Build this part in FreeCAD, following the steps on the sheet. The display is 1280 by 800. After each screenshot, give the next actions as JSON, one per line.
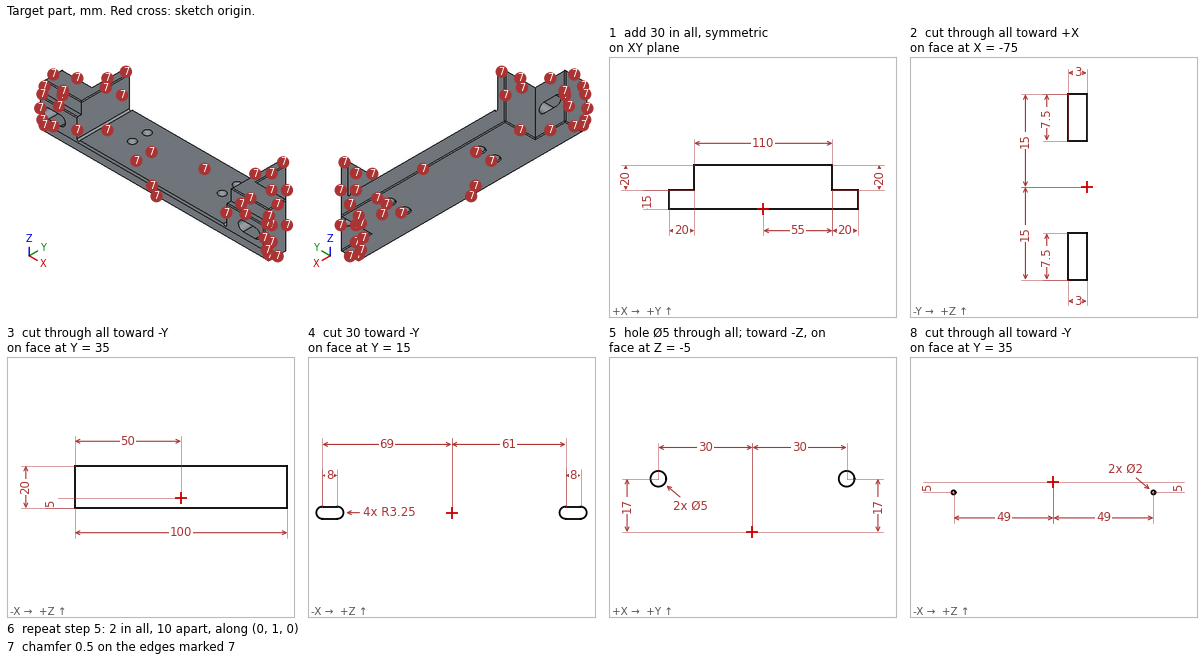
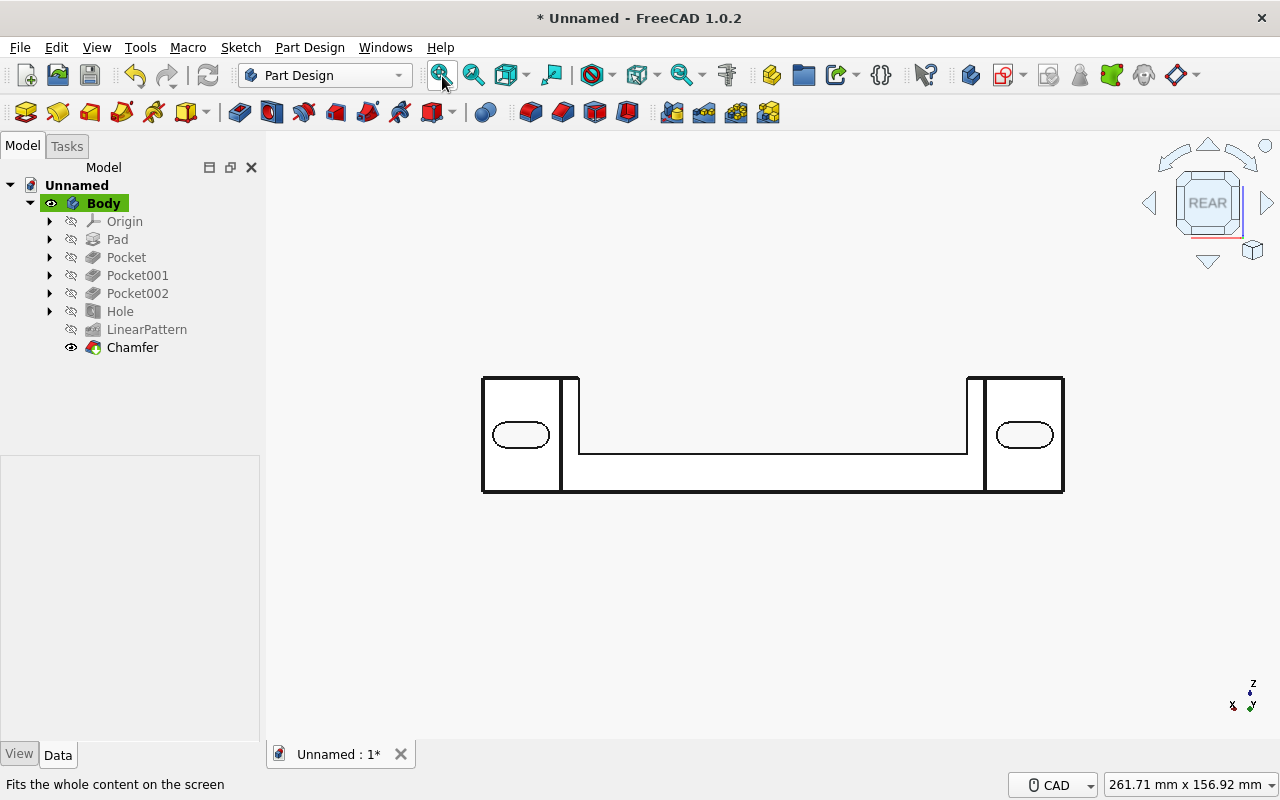
{"action": "left_click", "coordinate": [592, 466]}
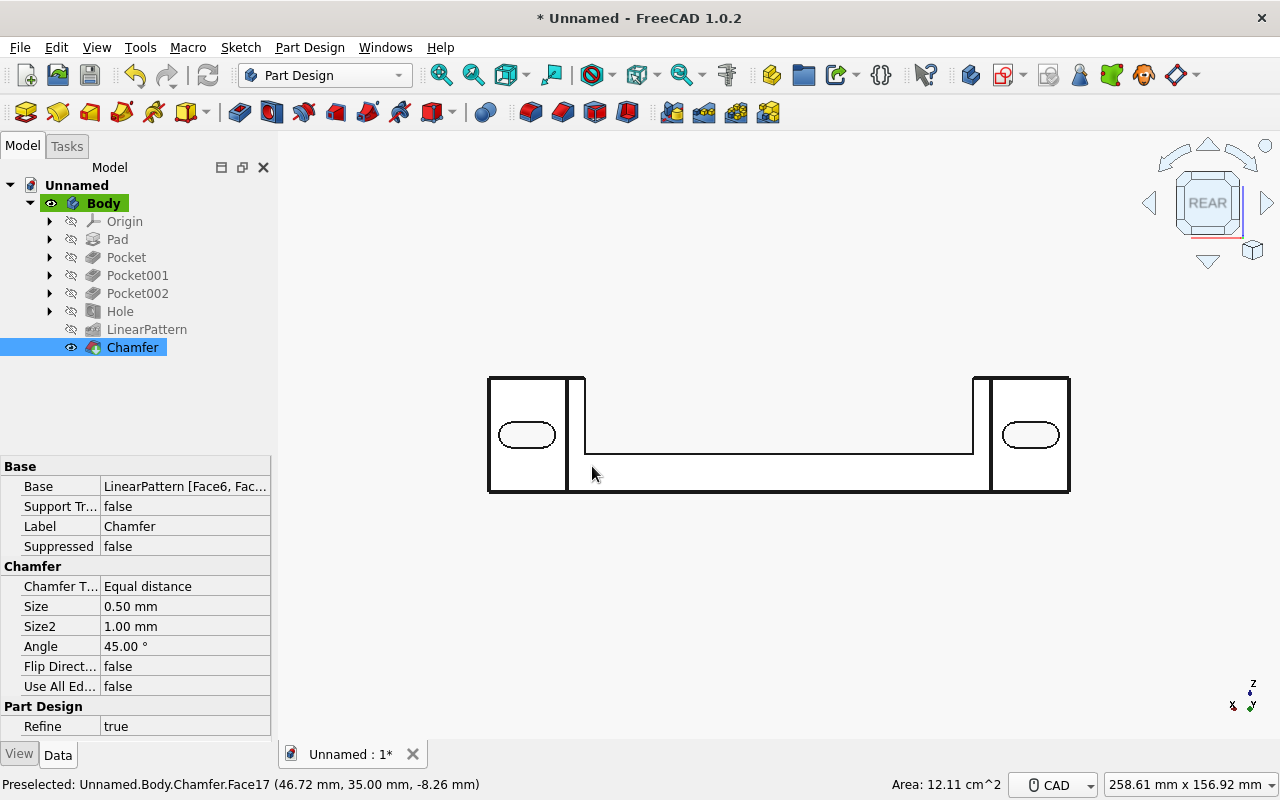
{"action": "left_click", "coordinate": [1004, 76]}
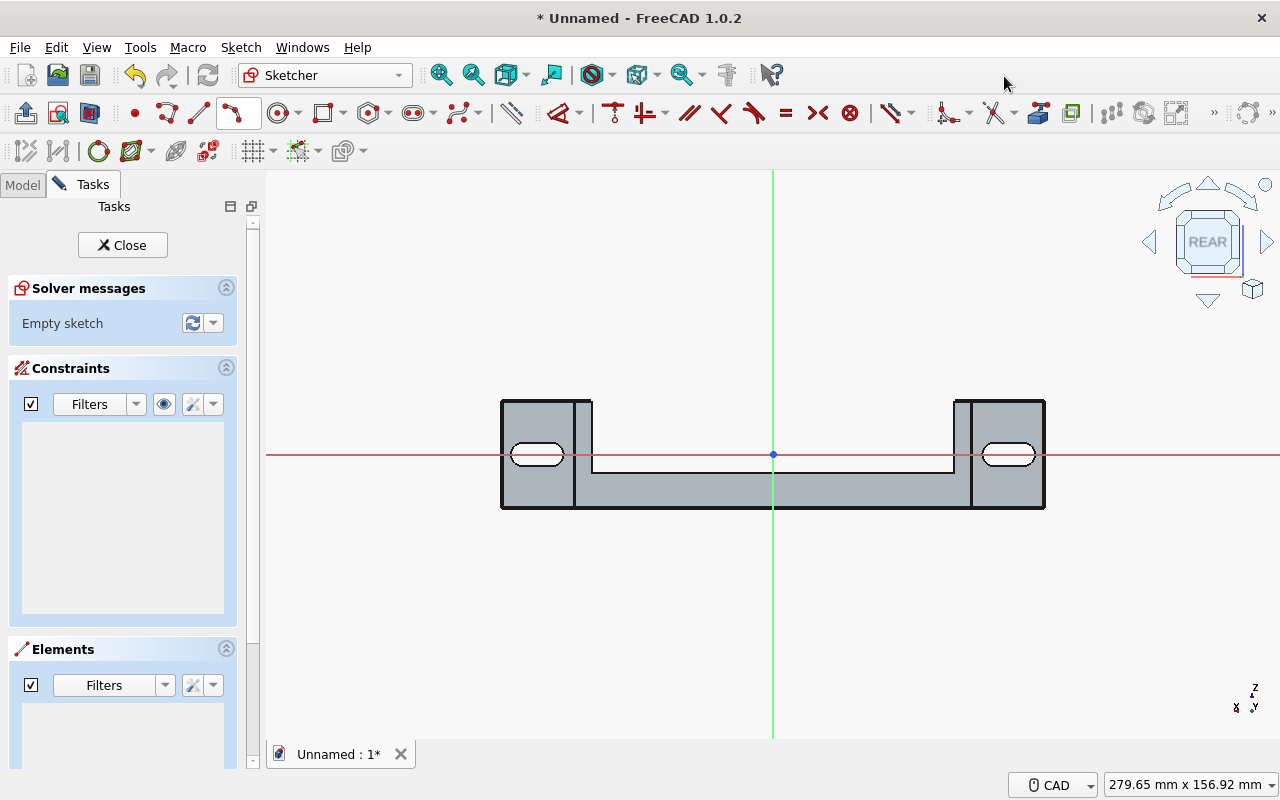
{"action": "scroll", "coordinate": [912, 487], "scroll_direction": "up", "scroll_amount": 2}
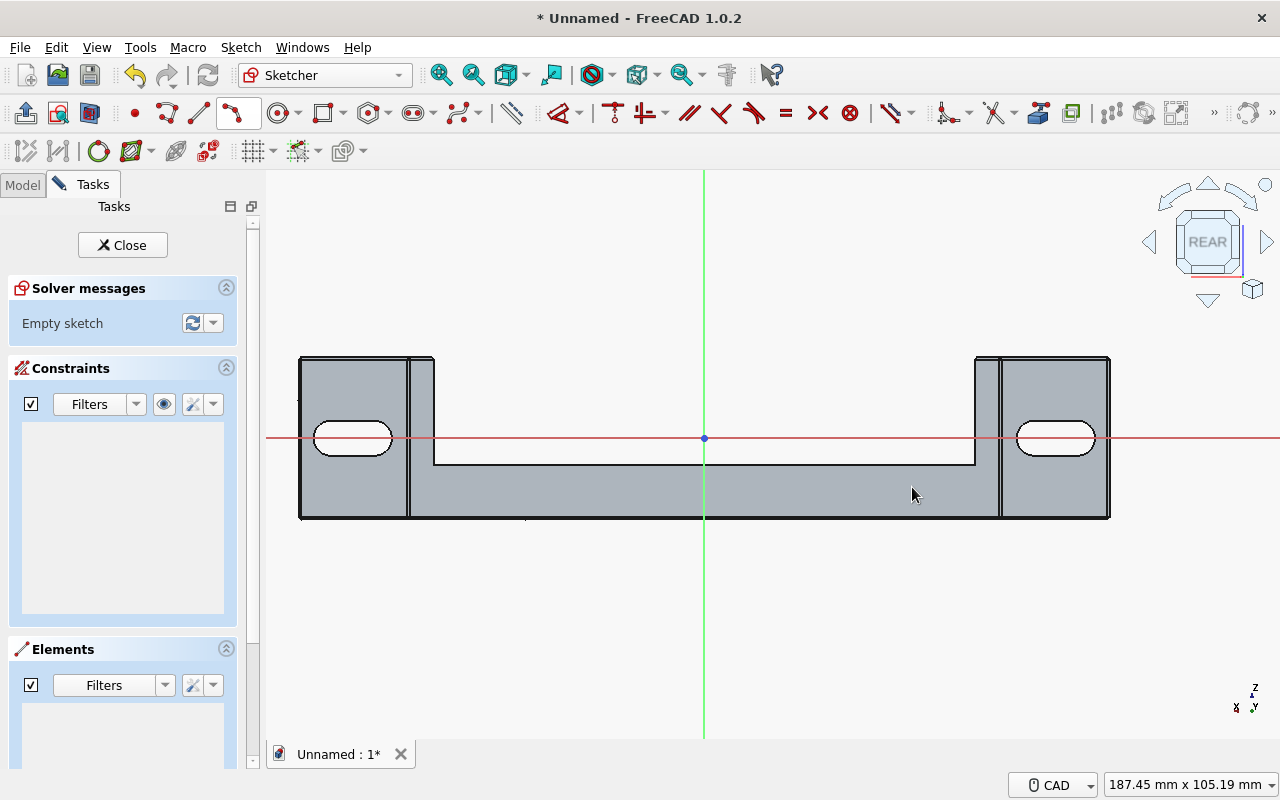
{"action": "key", "text": "g c"}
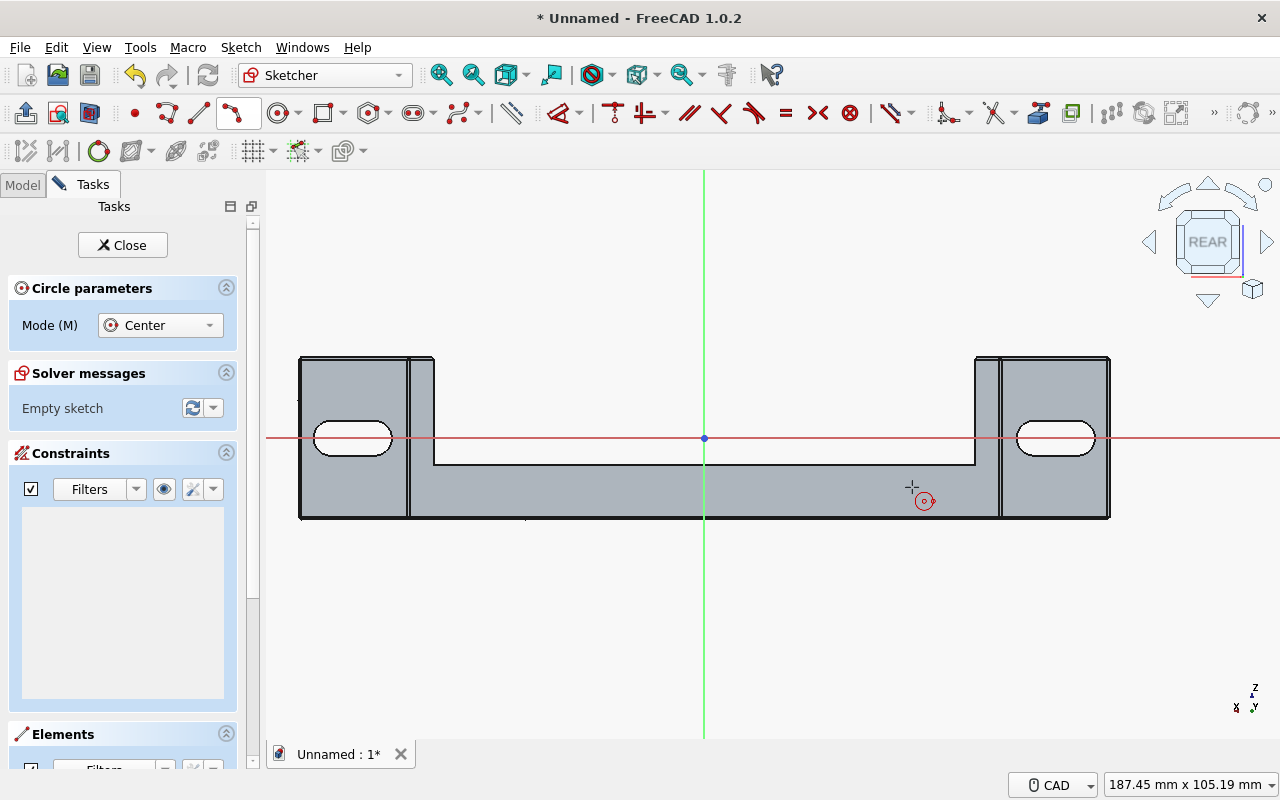
{"action": "scroll", "coordinate": [969, 465], "scroll_direction": "up", "scroll_amount": 8}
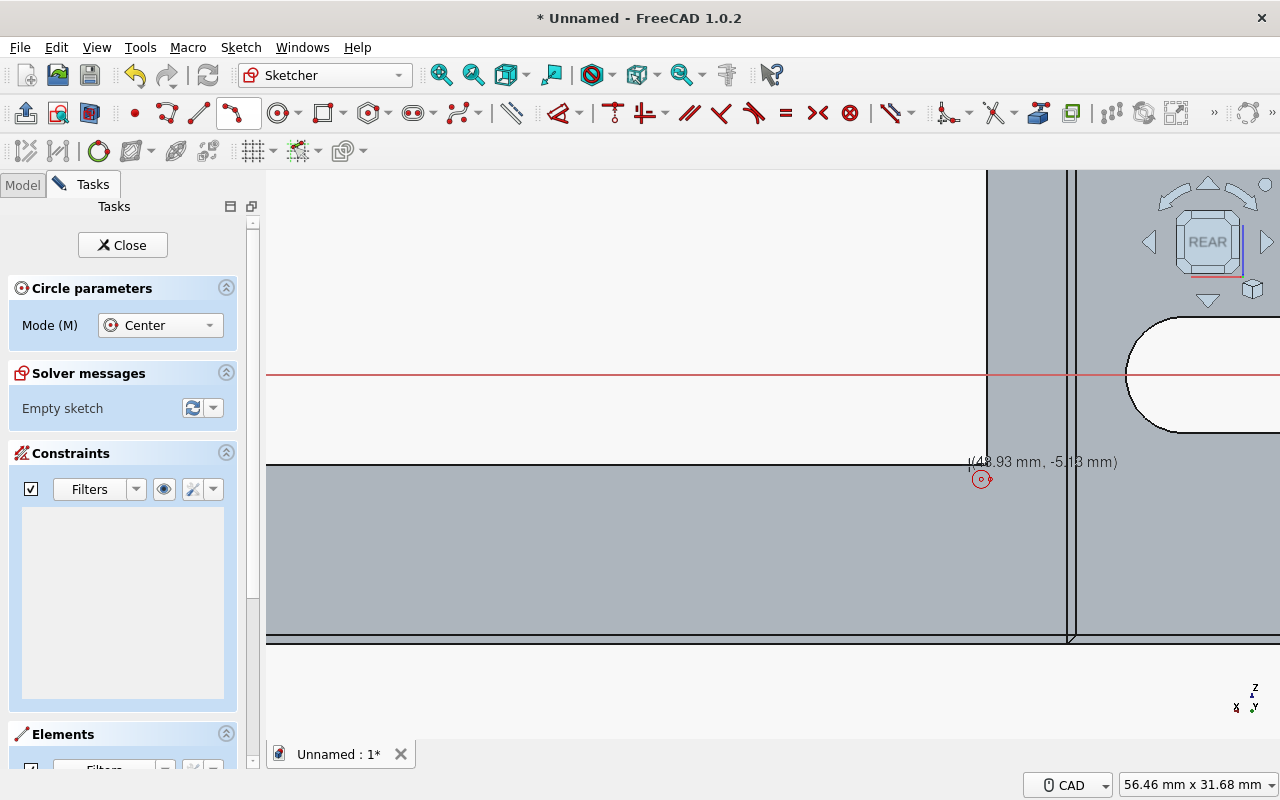
{"action": "scroll", "coordinate": [970, 466], "scroll_direction": "down", "scroll_amount": 8}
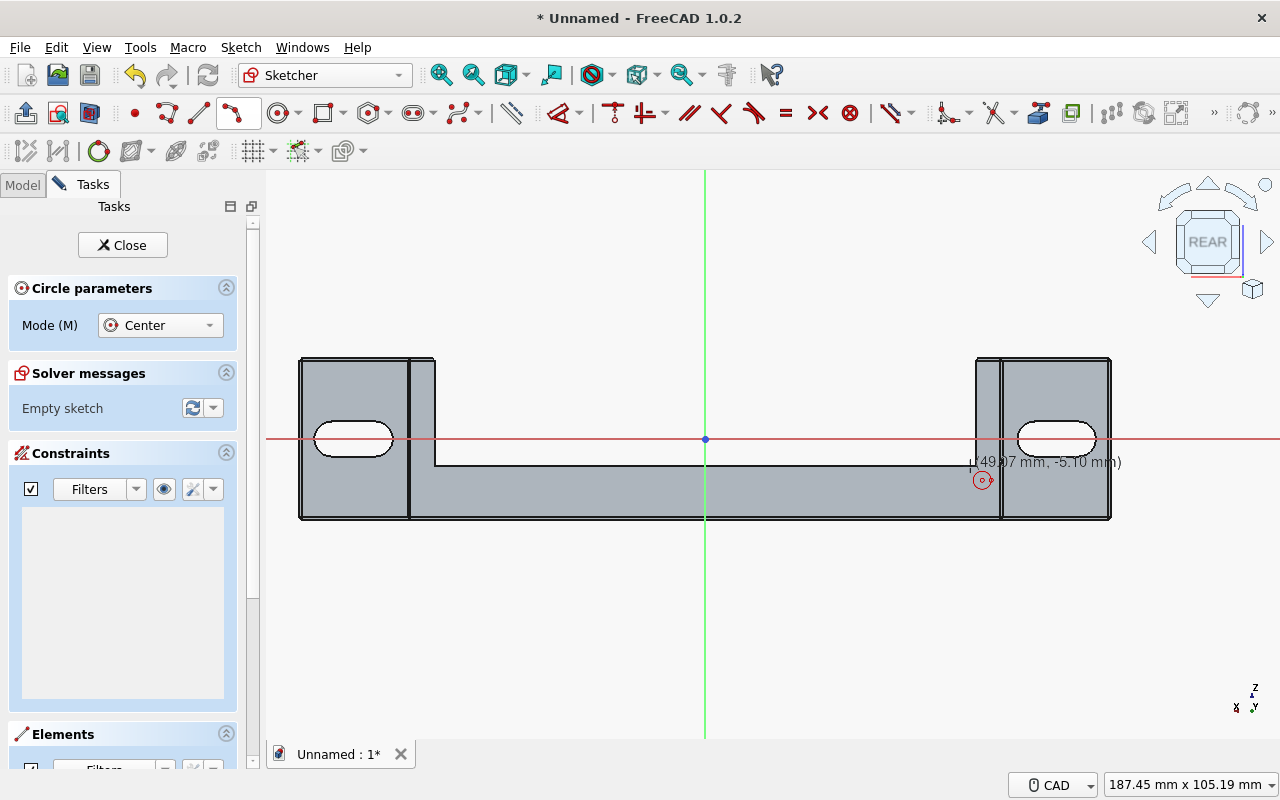
{"action": "left_click", "coordinate": [970, 466]}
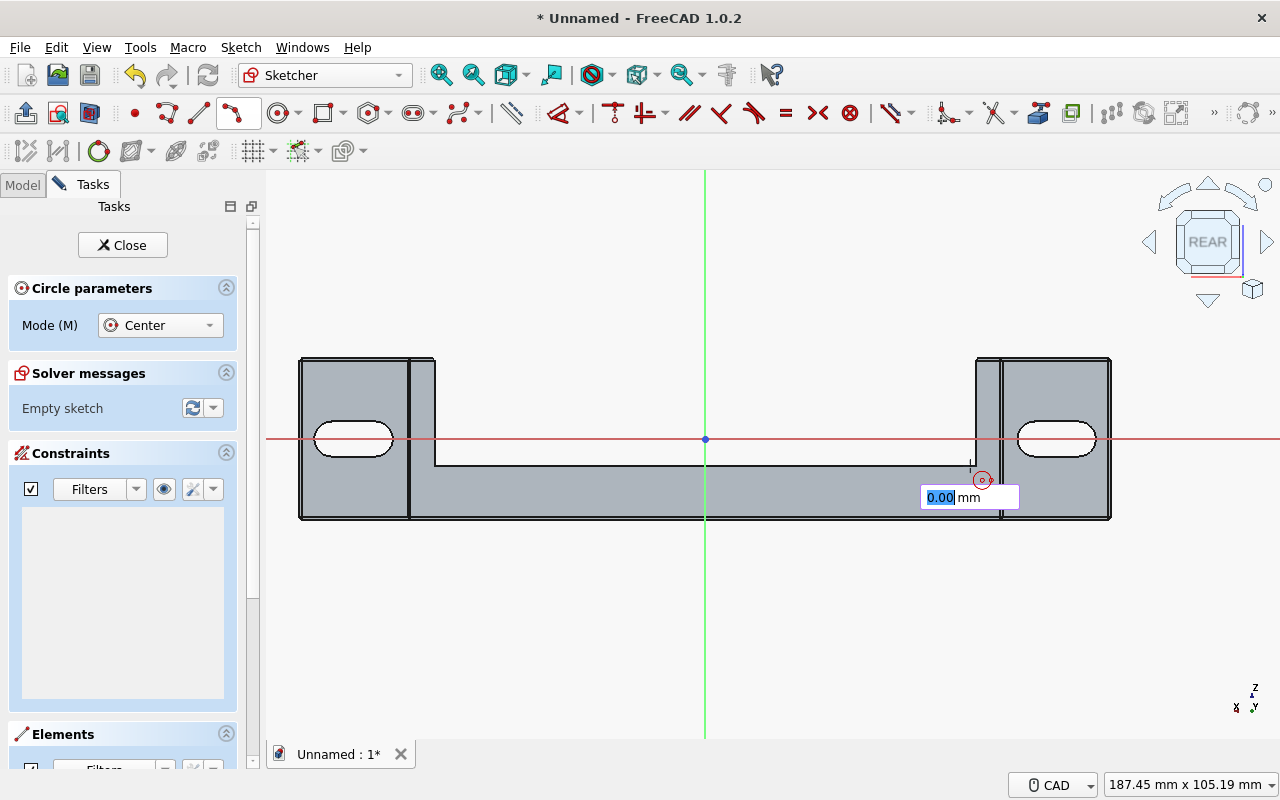
{"action": "scroll", "coordinate": [974, 462], "scroll_direction": "up", "scroll_amount": 6}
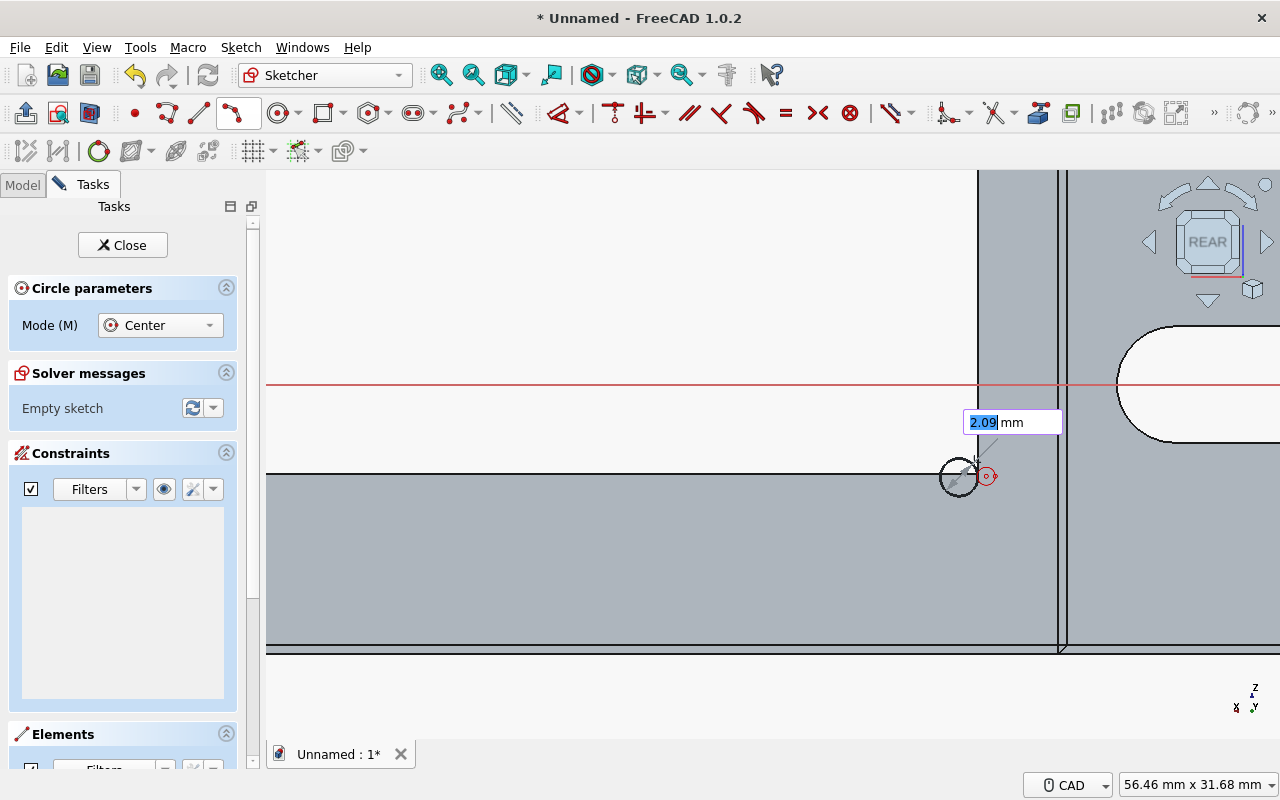
{"action": "left_click", "coordinate": [972, 462]}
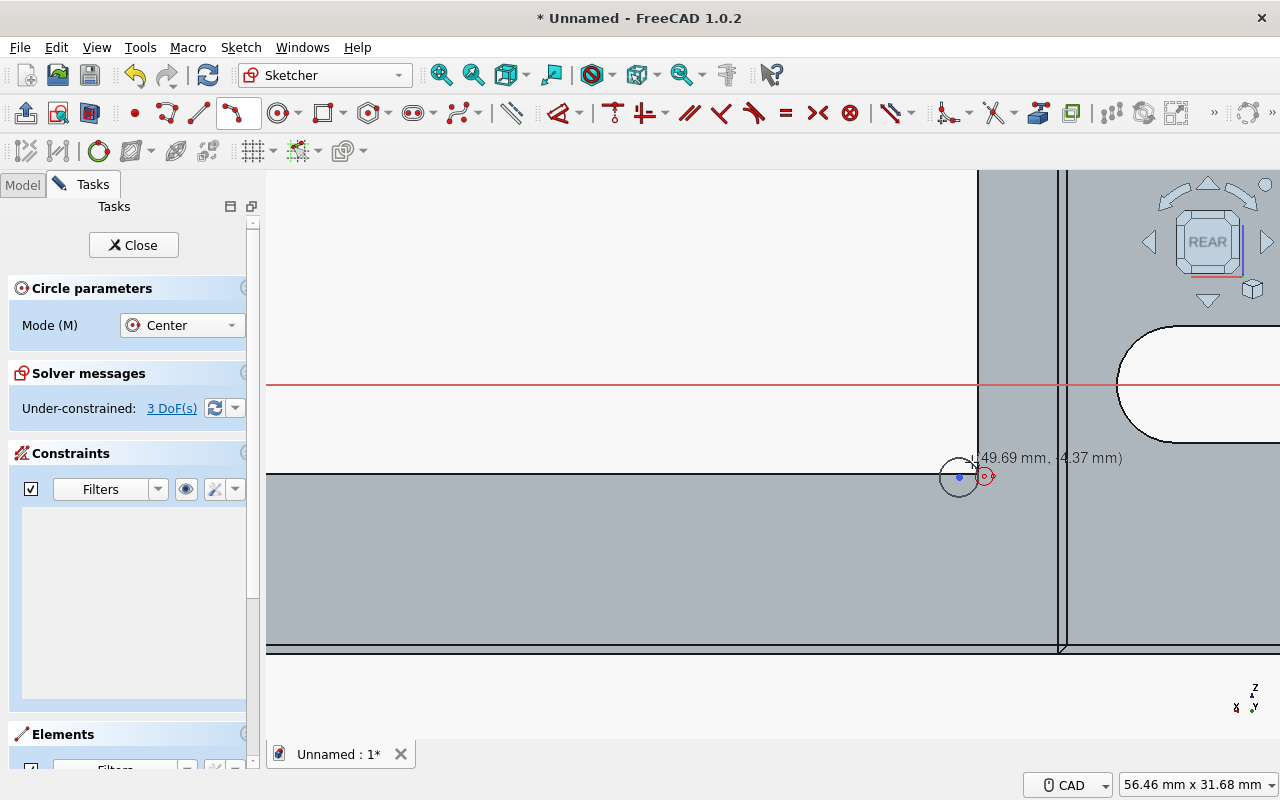
{"action": "scroll", "coordinate": [974, 461], "scroll_direction": "down", "scroll_amount": 6}